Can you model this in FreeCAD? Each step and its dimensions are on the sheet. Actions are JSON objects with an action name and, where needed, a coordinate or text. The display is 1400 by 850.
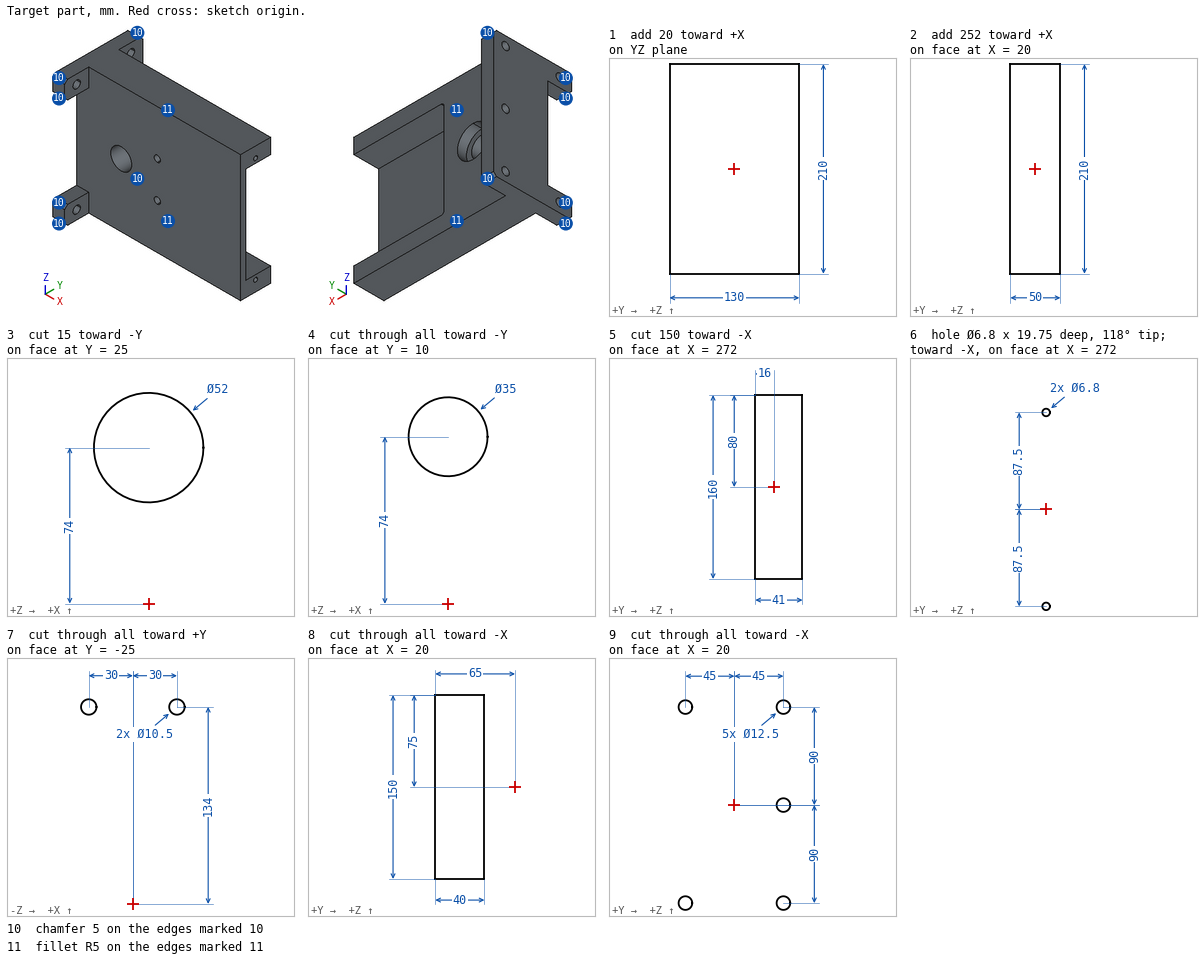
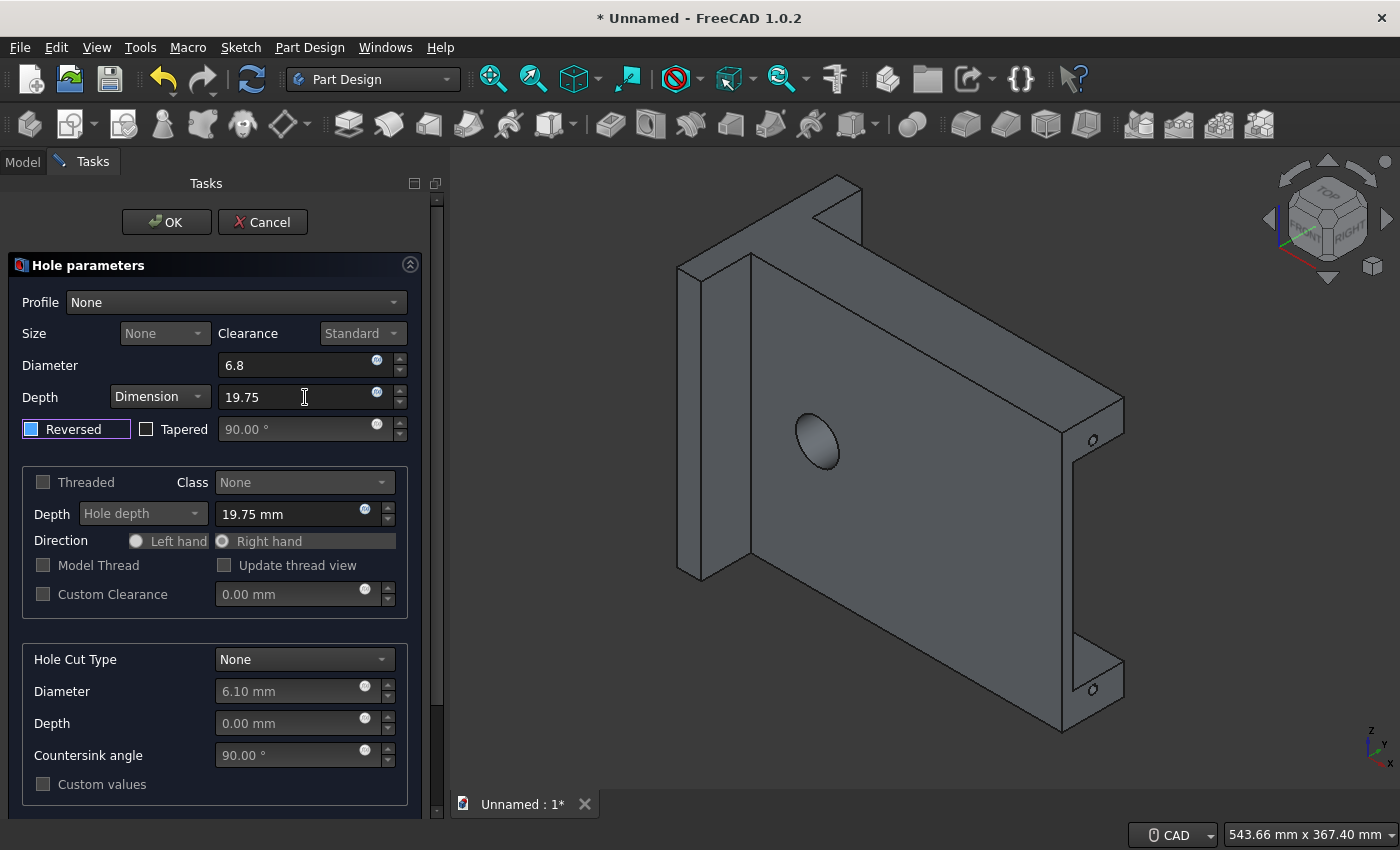
{"action": "left_click", "coordinate": [167, 222]}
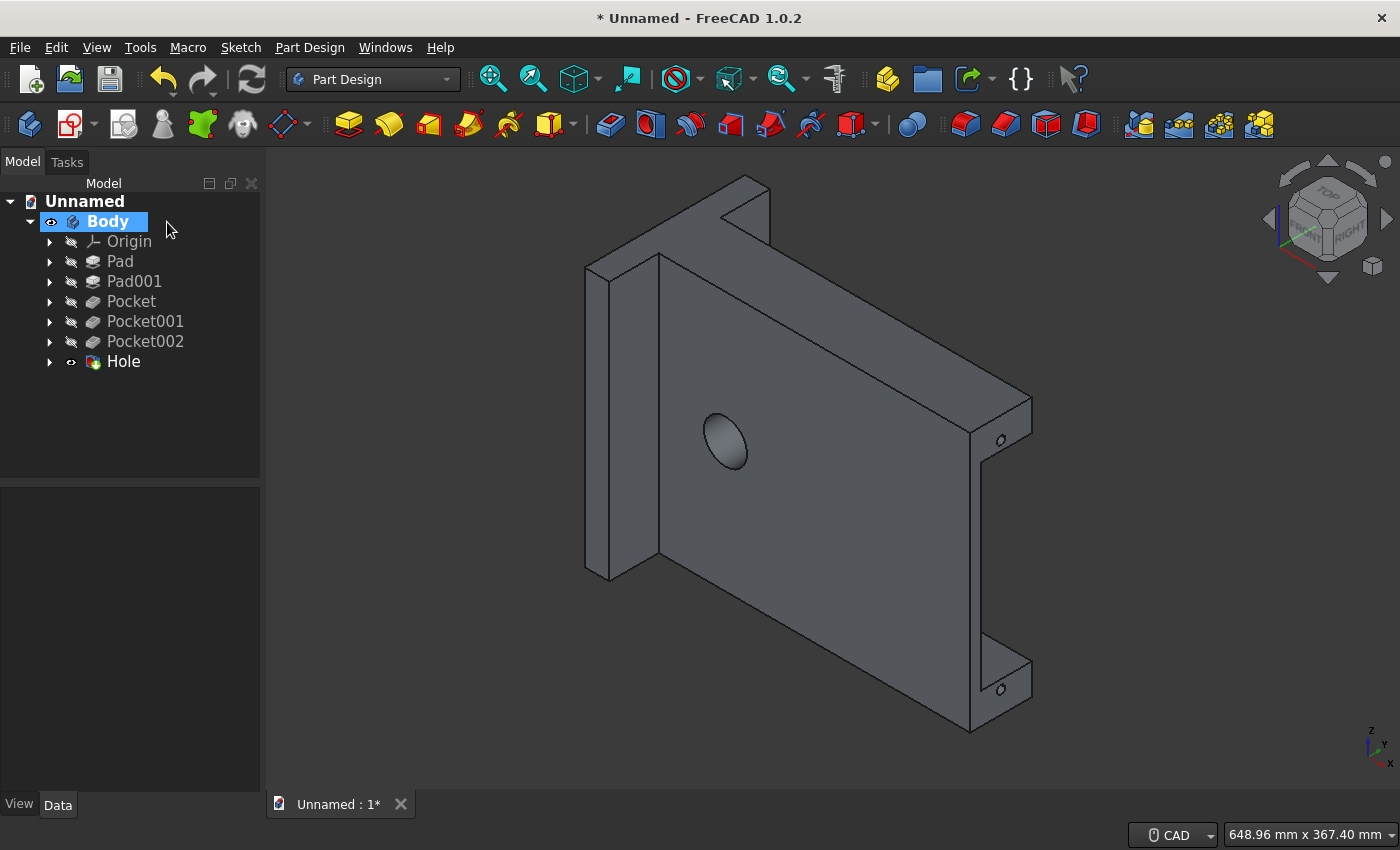
{"action": "left_click", "coordinate": [859, 518]}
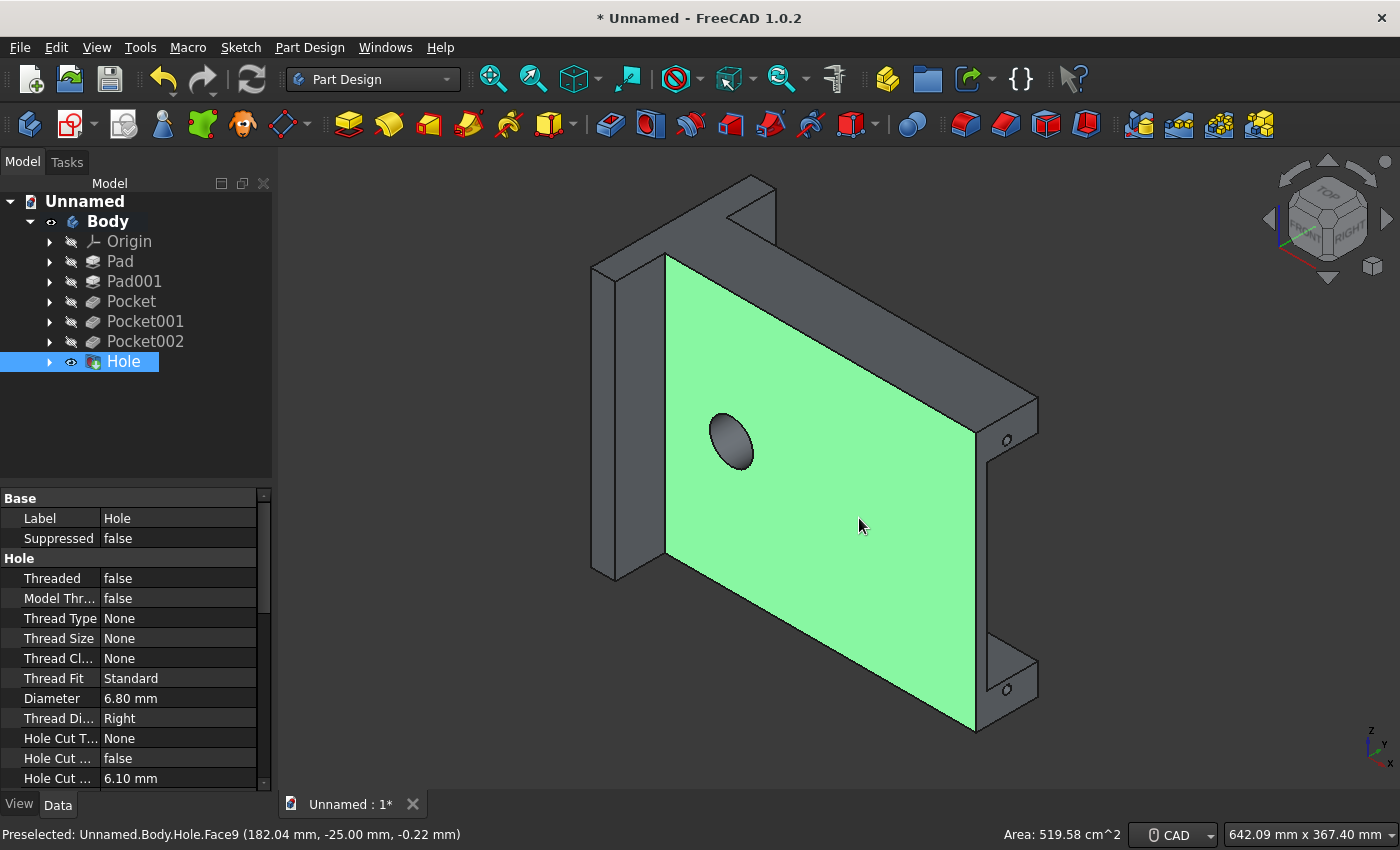
{"action": "left_click", "coordinate": [70, 124]}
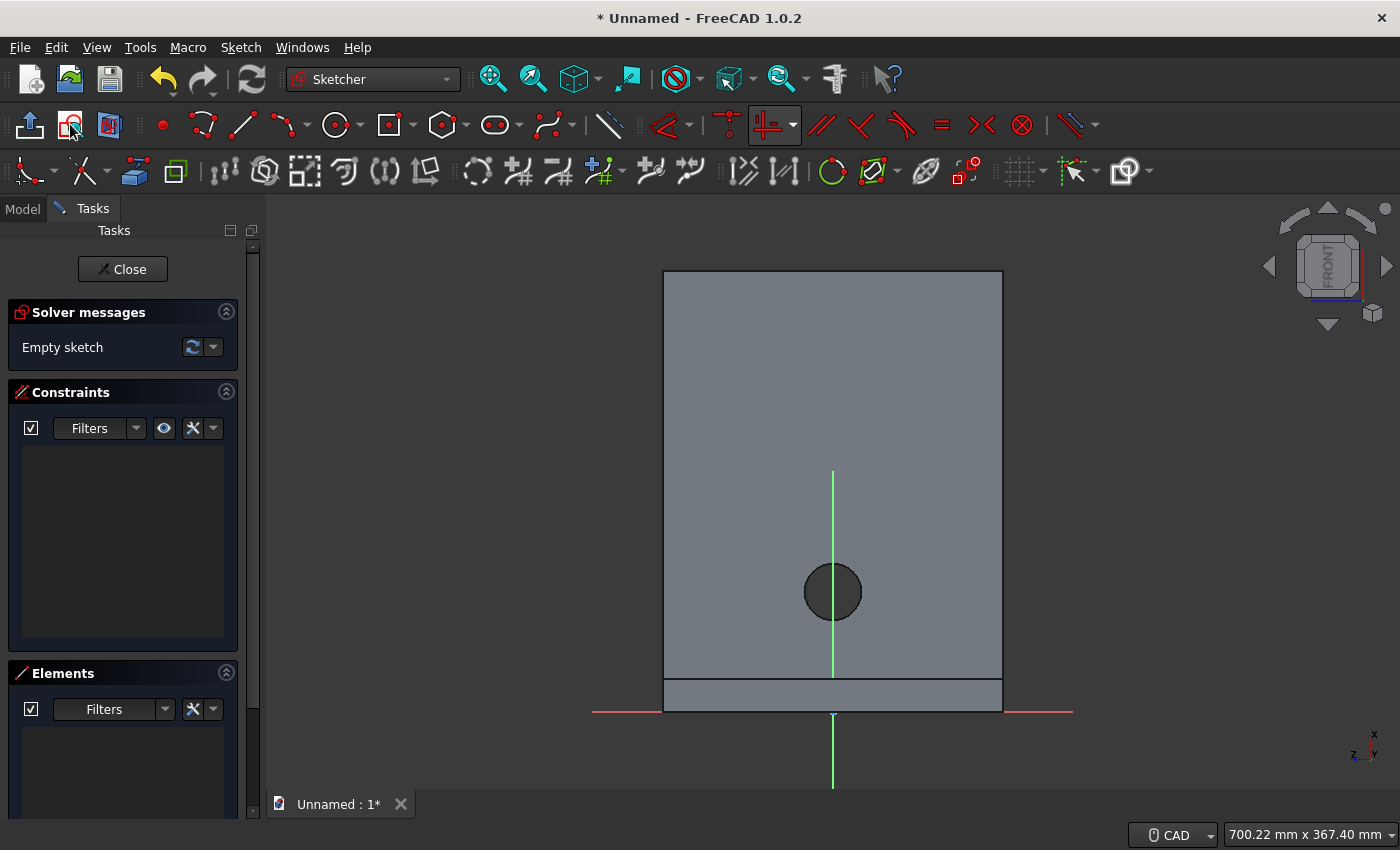
{"action": "scroll", "coordinate": [916, 730], "scroll_direction": "up", "scroll_amount": 3}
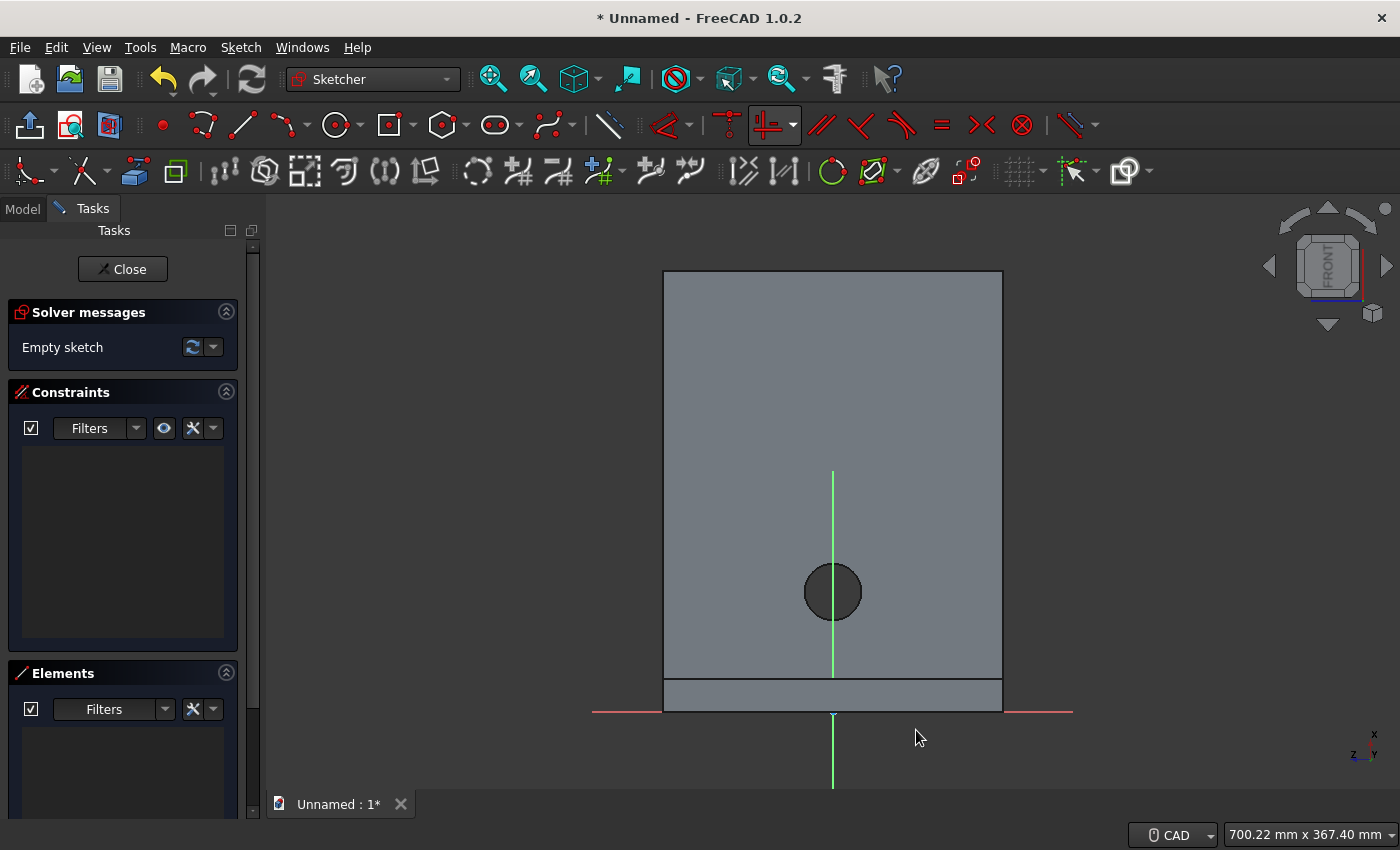
{"action": "left_click", "coordinate": [336, 126]}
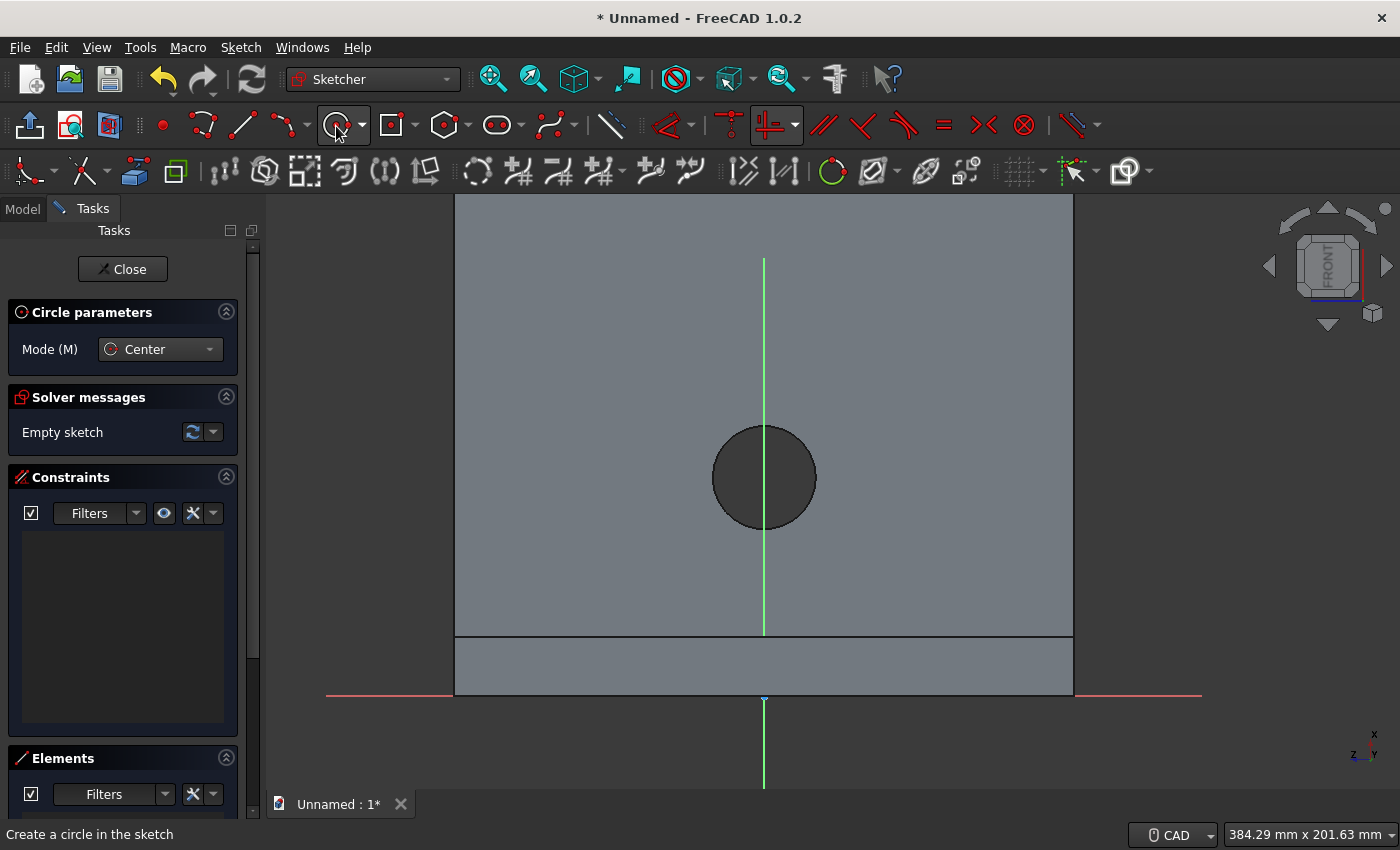
{"action": "scroll", "coordinate": [853, 301], "scroll_direction": "up", "scroll_amount": 2}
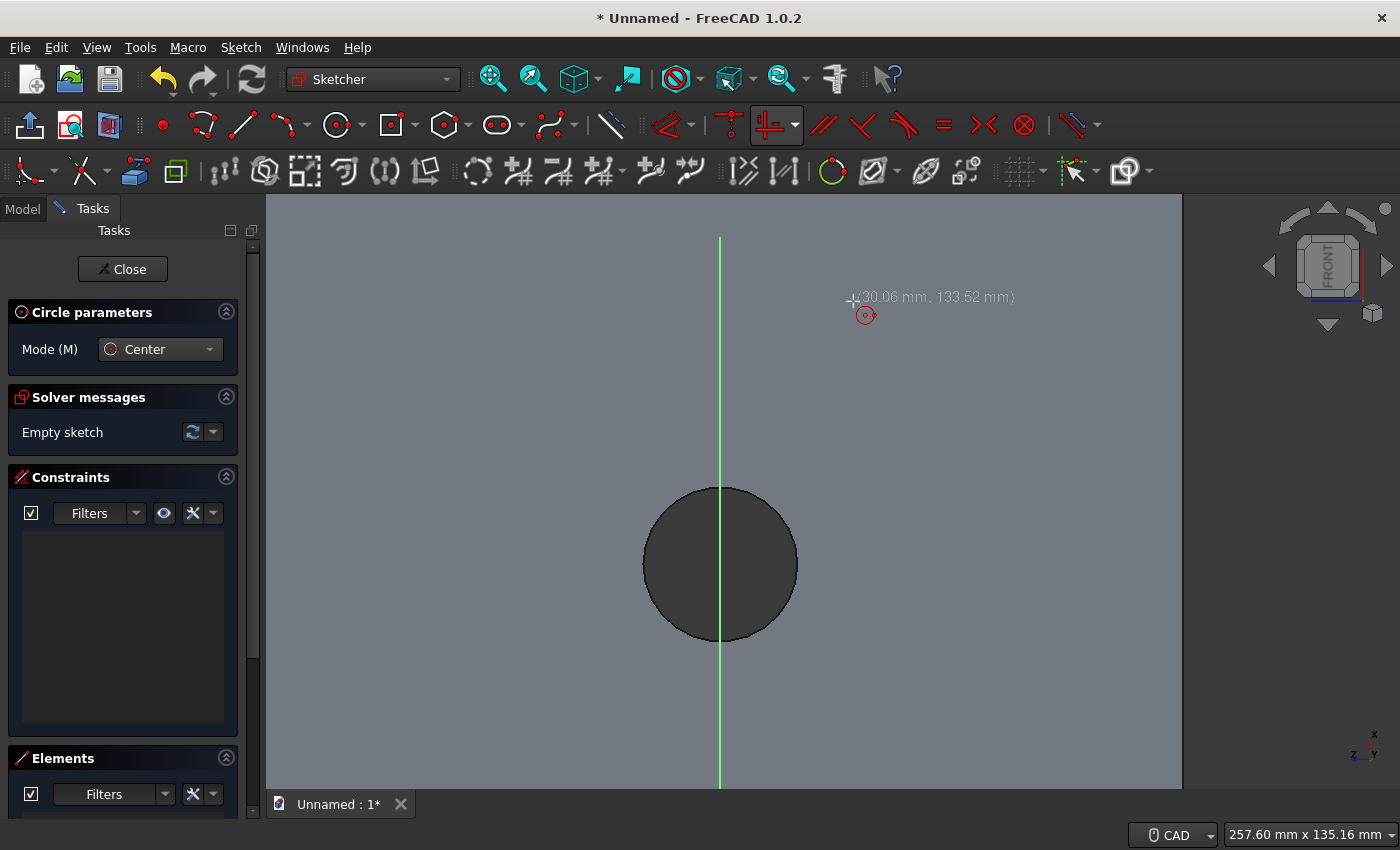
{"action": "left_click", "coordinate": [852, 300]}
{"action": "left_click", "coordinate": [869, 284]}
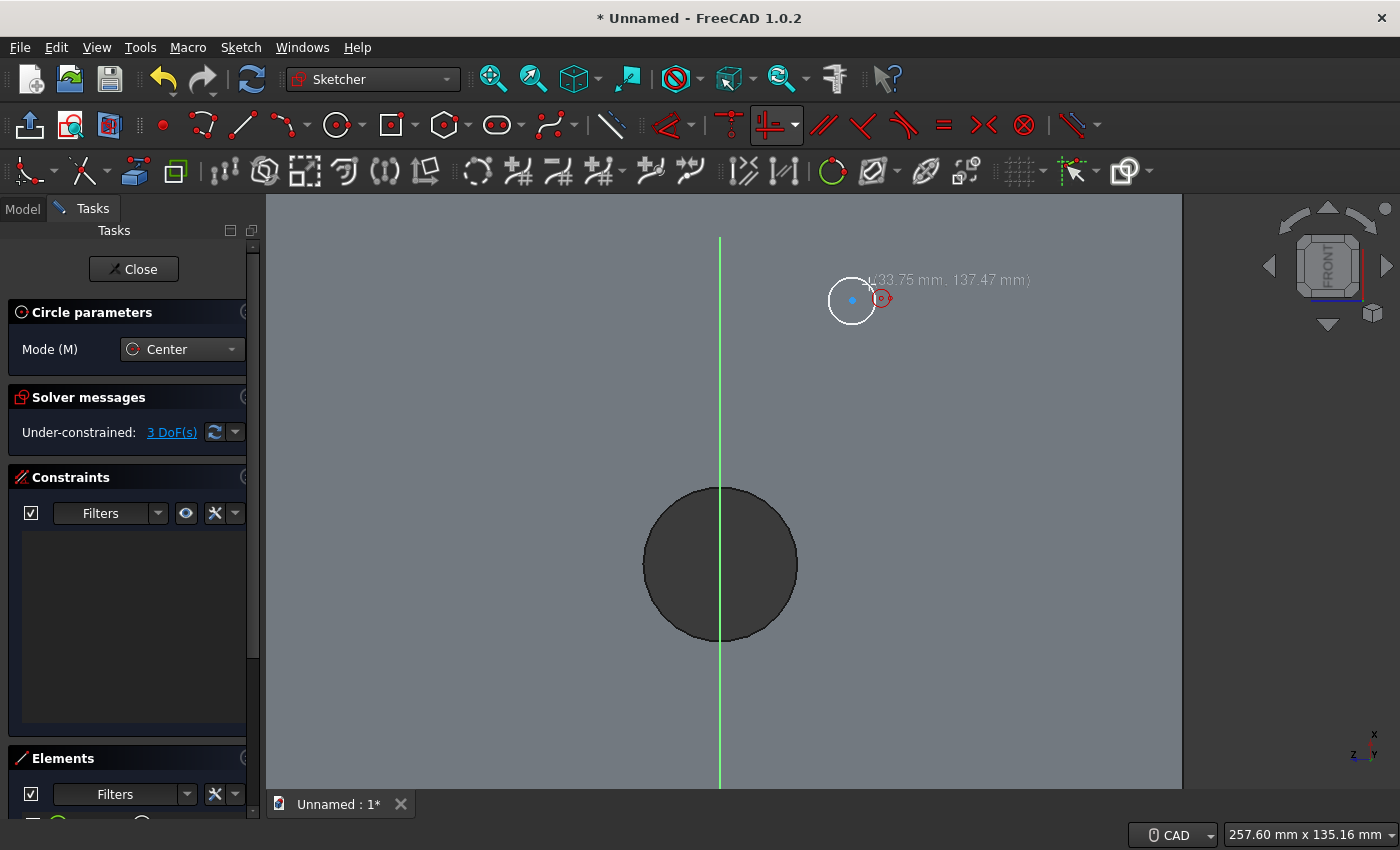
{"action": "left_click", "coordinate": [588, 300]}
{"action": "left_click", "coordinate": [605, 284]}
{"action": "key", "text": "Escape"}